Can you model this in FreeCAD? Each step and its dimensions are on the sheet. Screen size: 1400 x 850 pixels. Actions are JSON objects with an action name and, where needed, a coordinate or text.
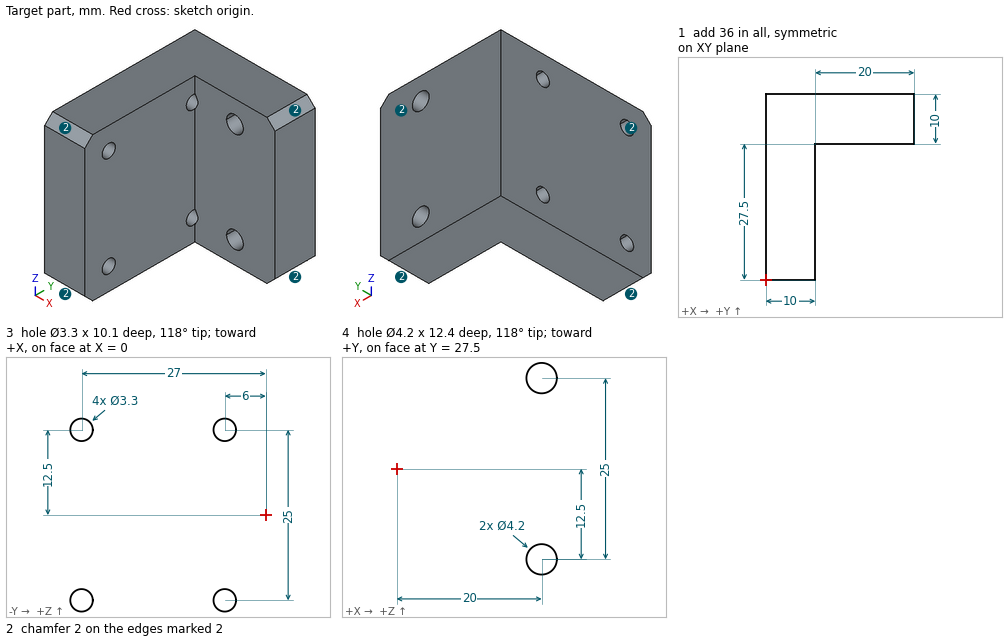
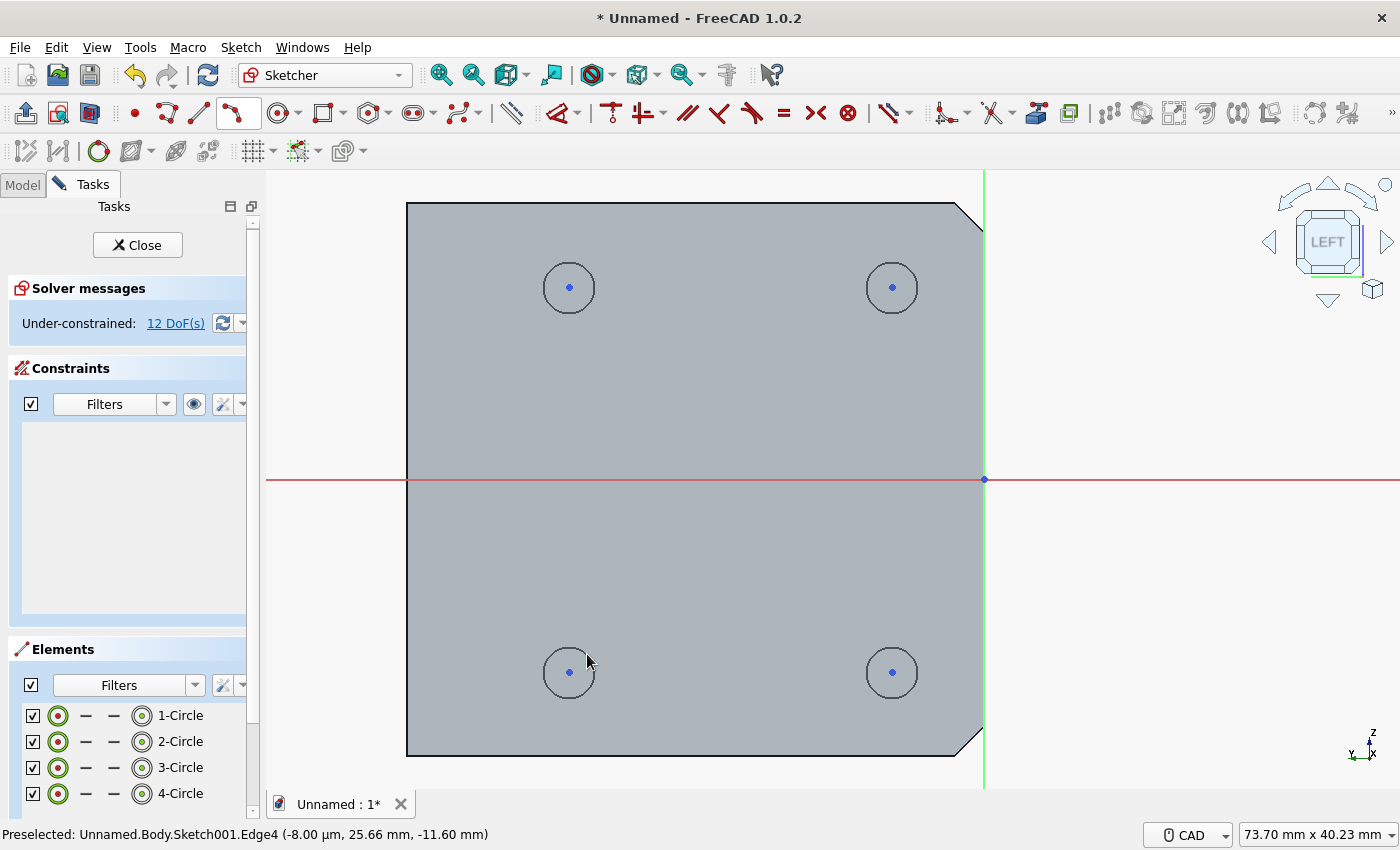
{"action": "left_click", "coordinate": [587, 270]}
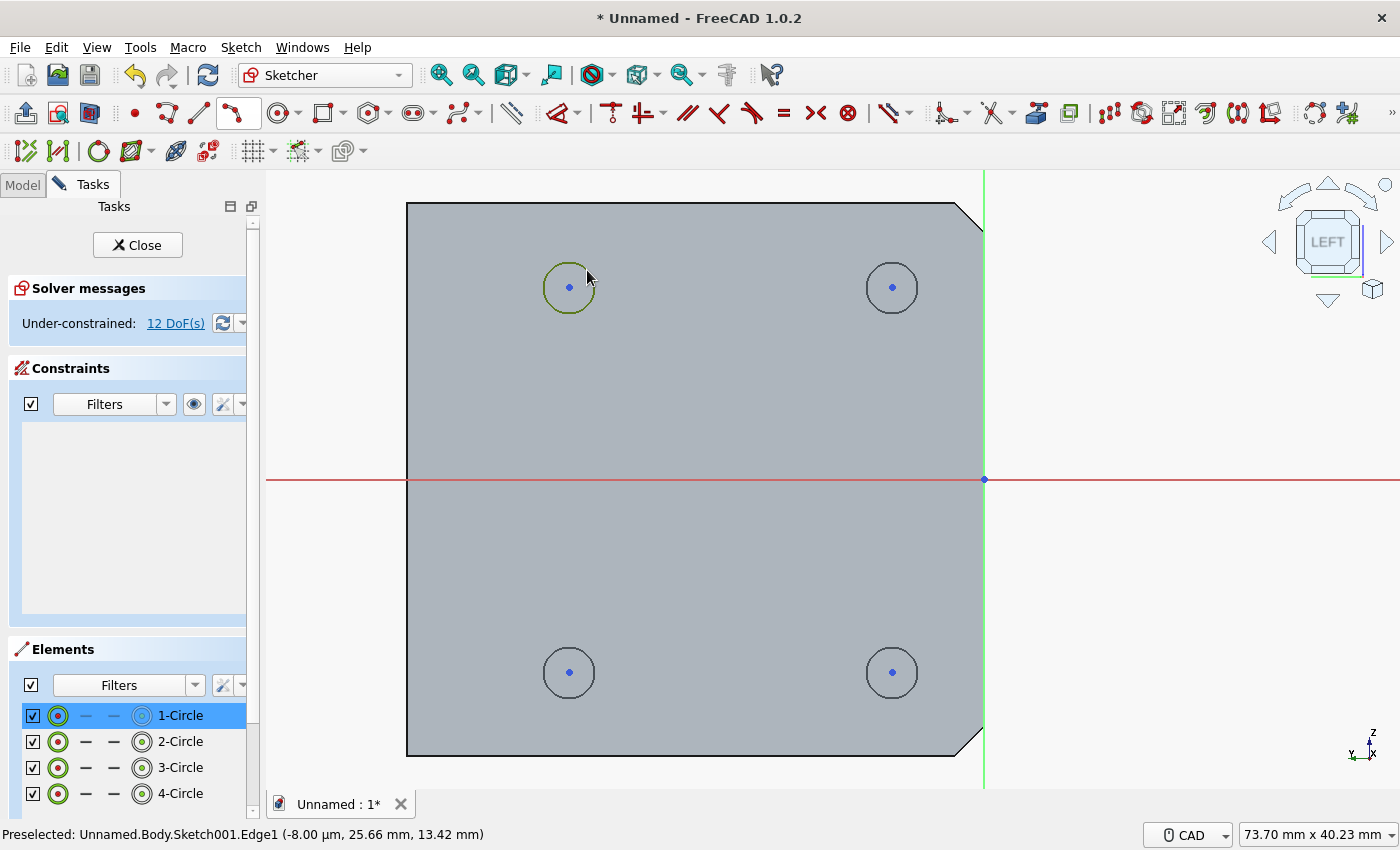
{"action": "left_click", "coordinate": [910, 270]}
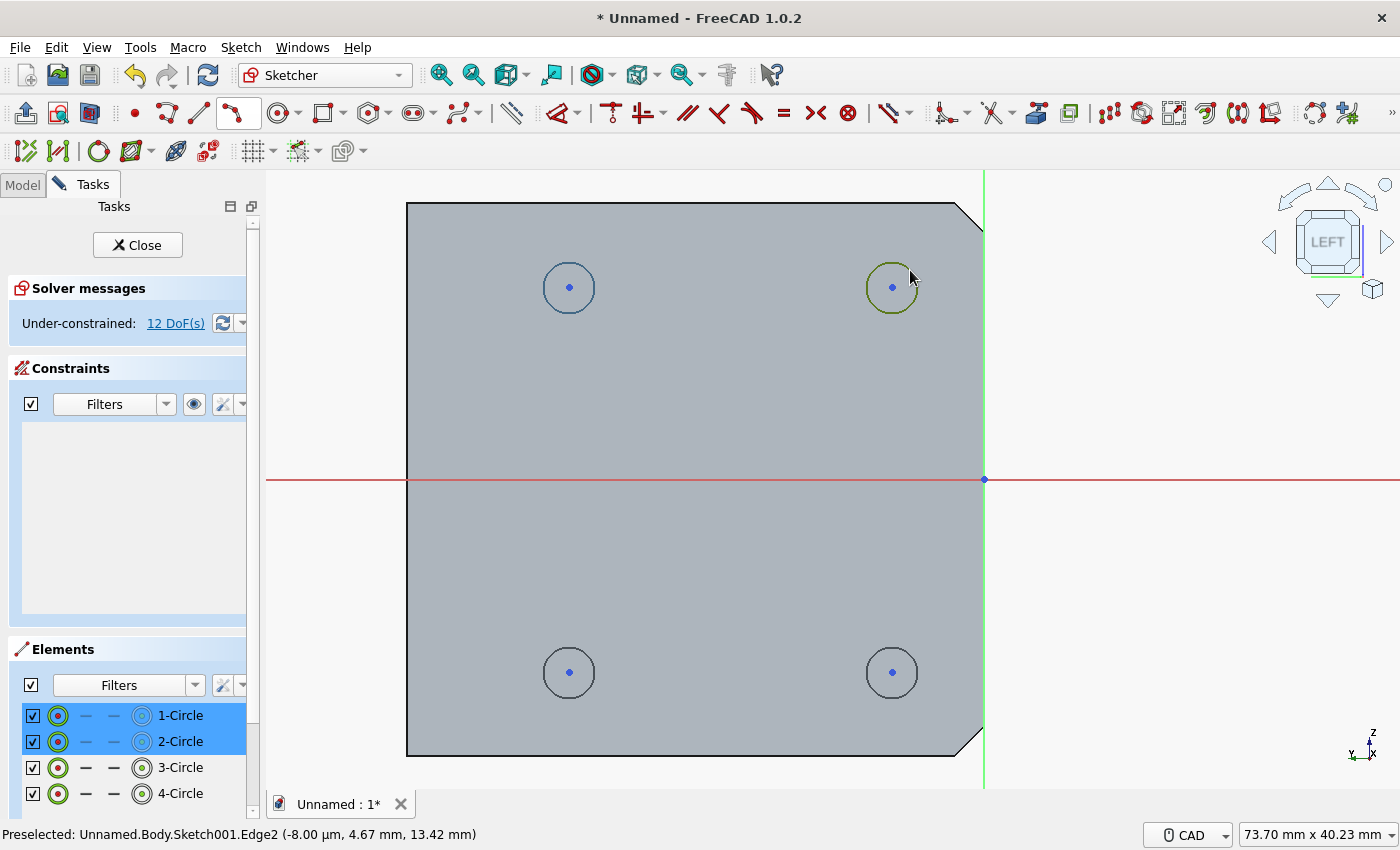
{"action": "left_click", "coordinate": [910, 655]}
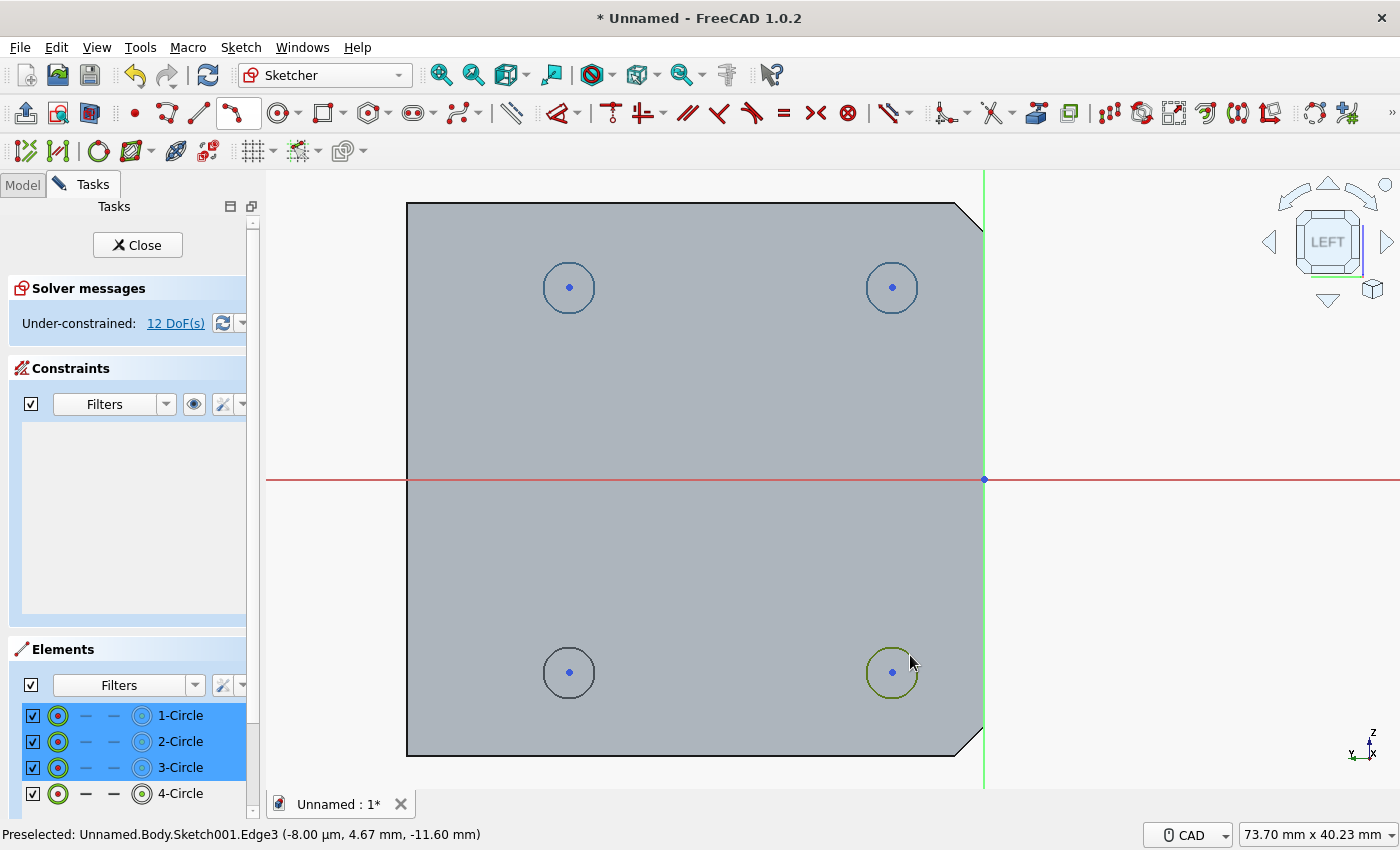
{"action": "left_click", "coordinate": [587, 655]}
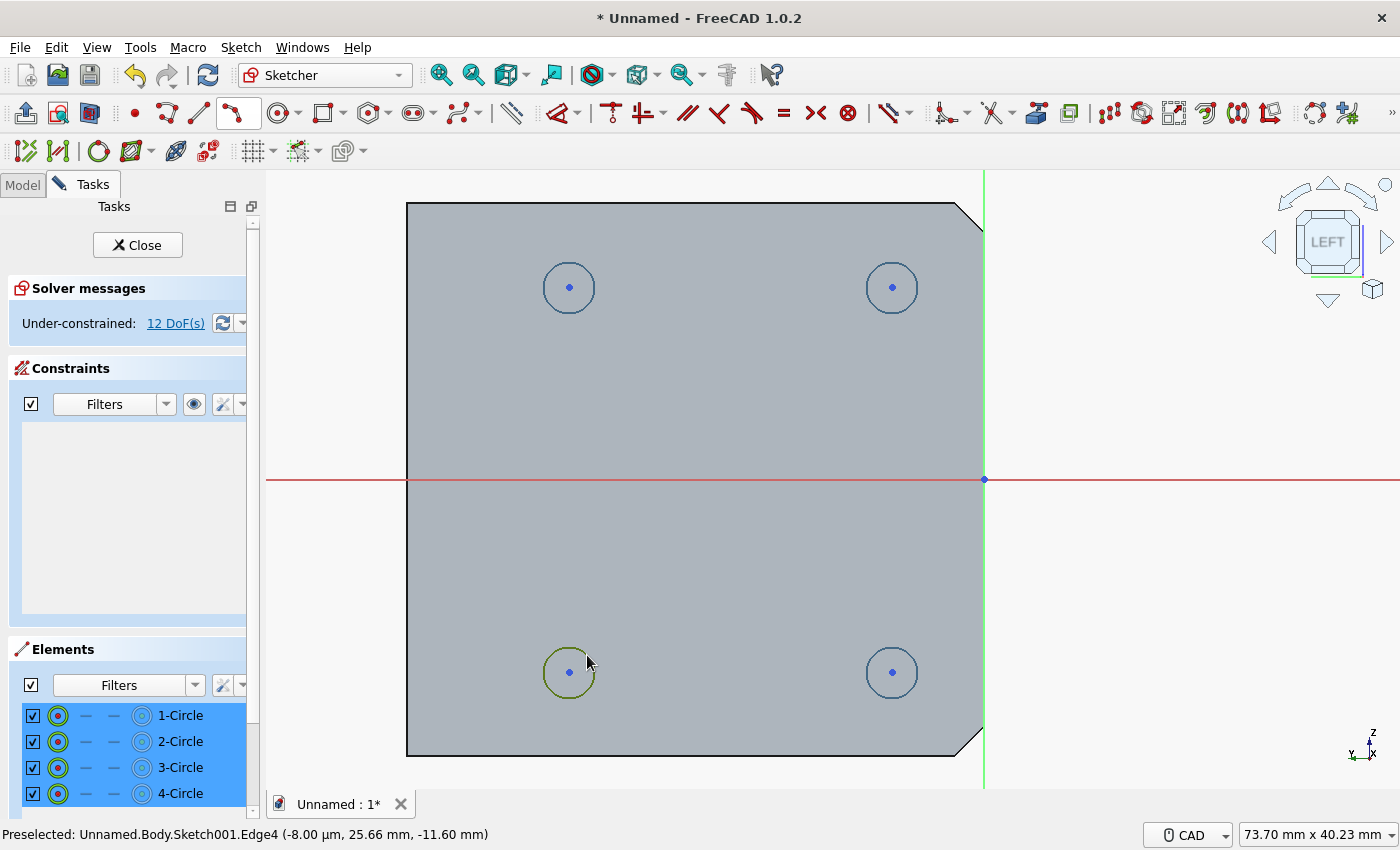
{"action": "key", "text": "e"}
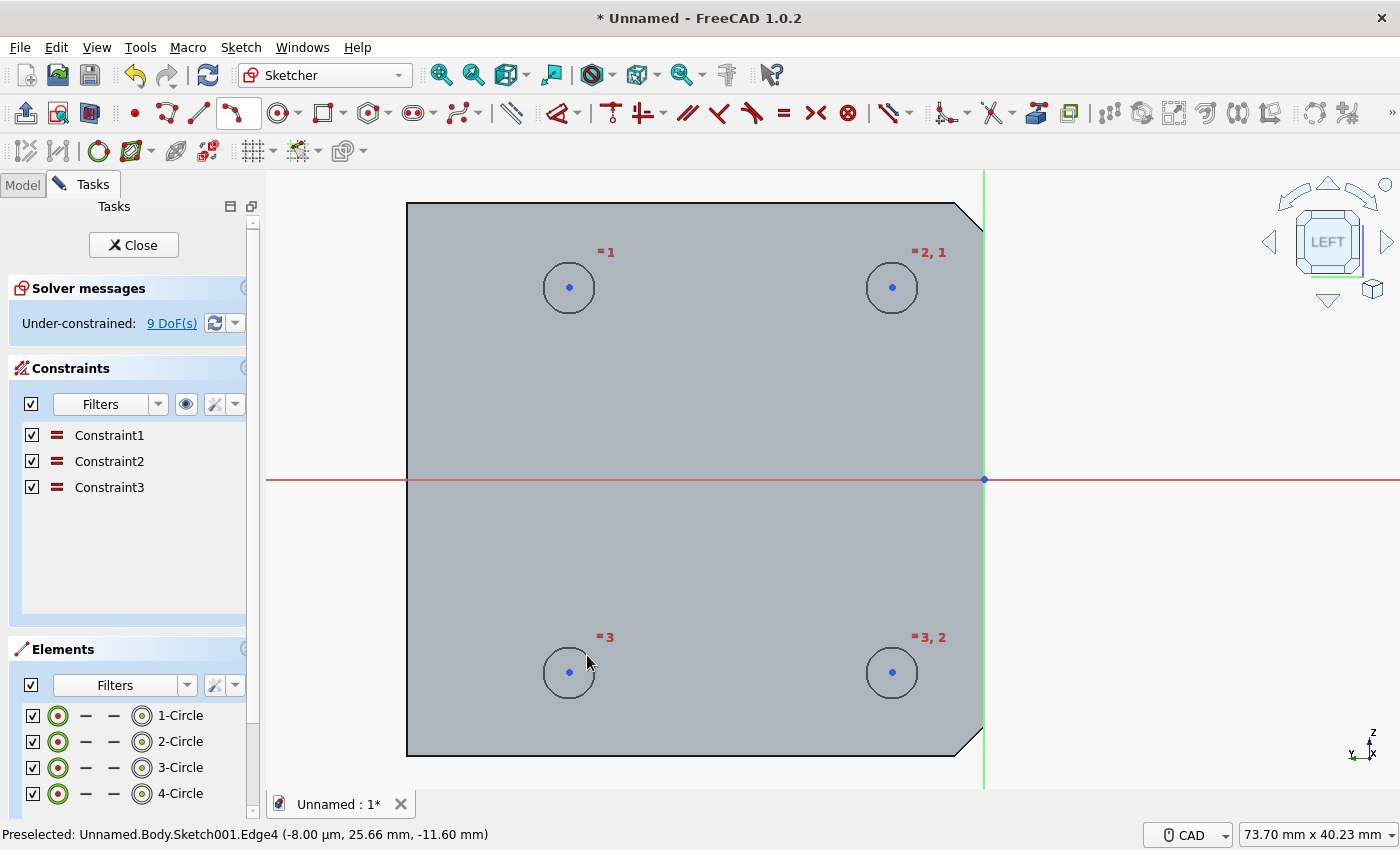
{"action": "left_click", "coordinate": [569, 288]}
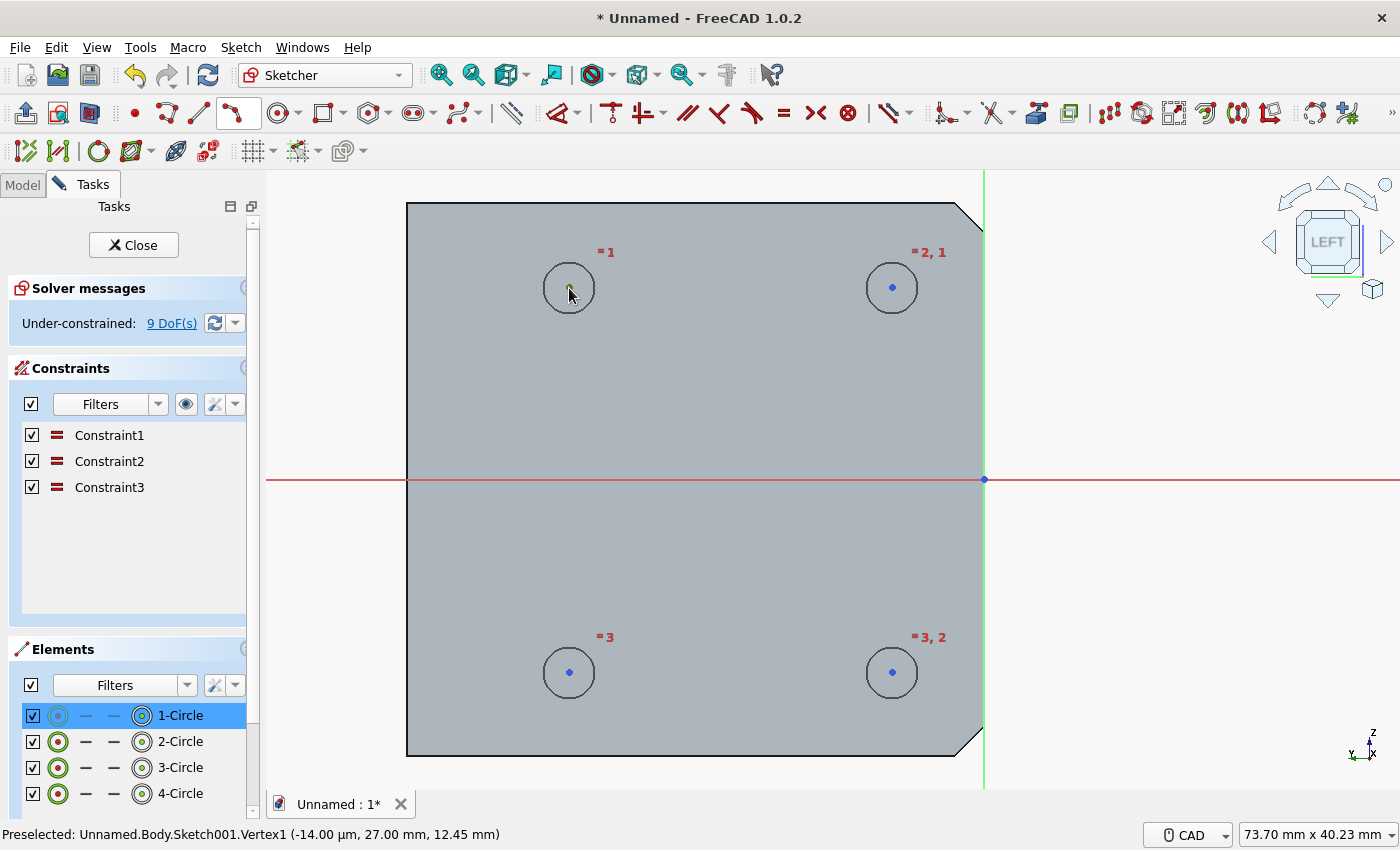
{"action": "left_click", "coordinate": [892, 288]}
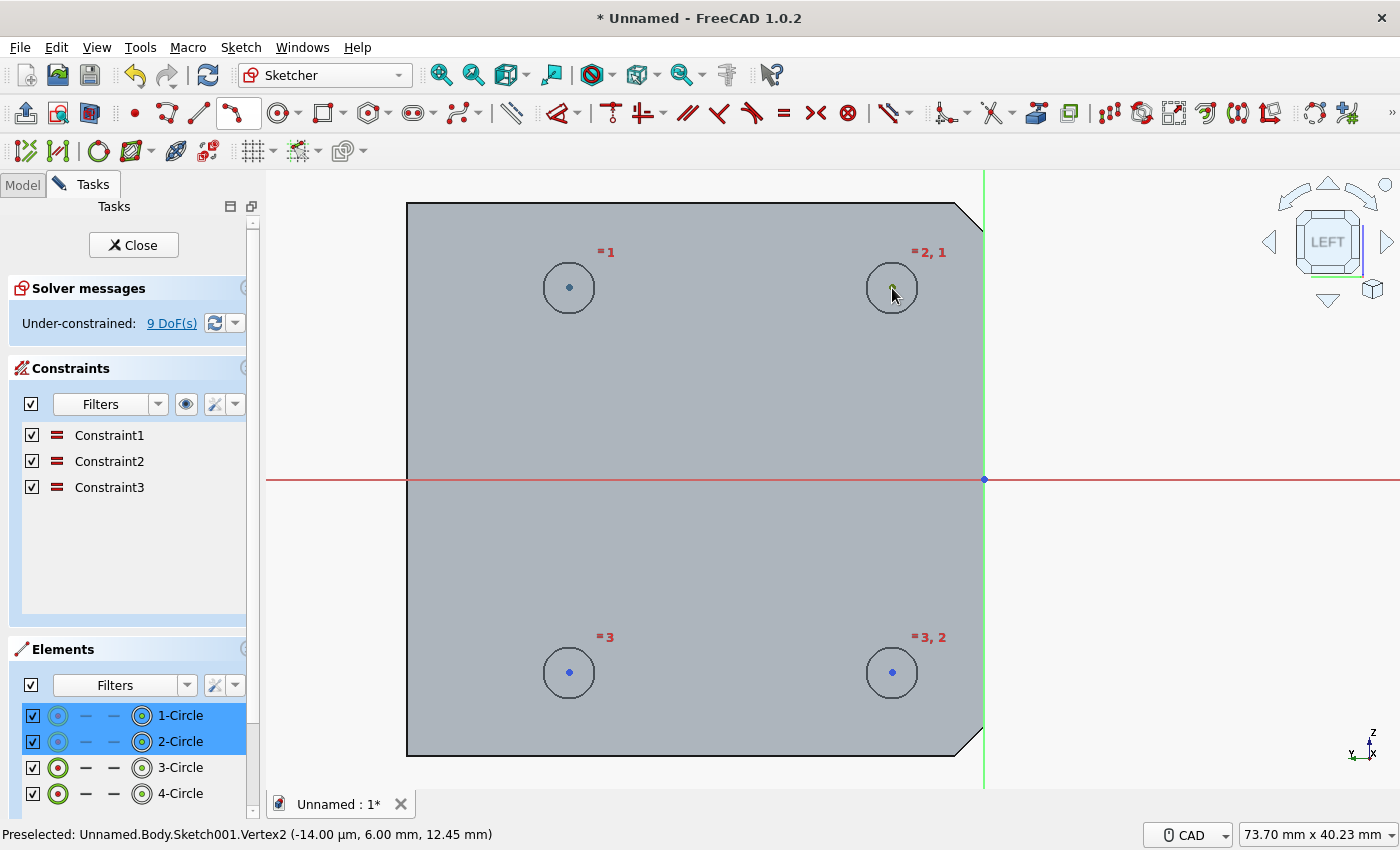
{"action": "key", "text": "h"}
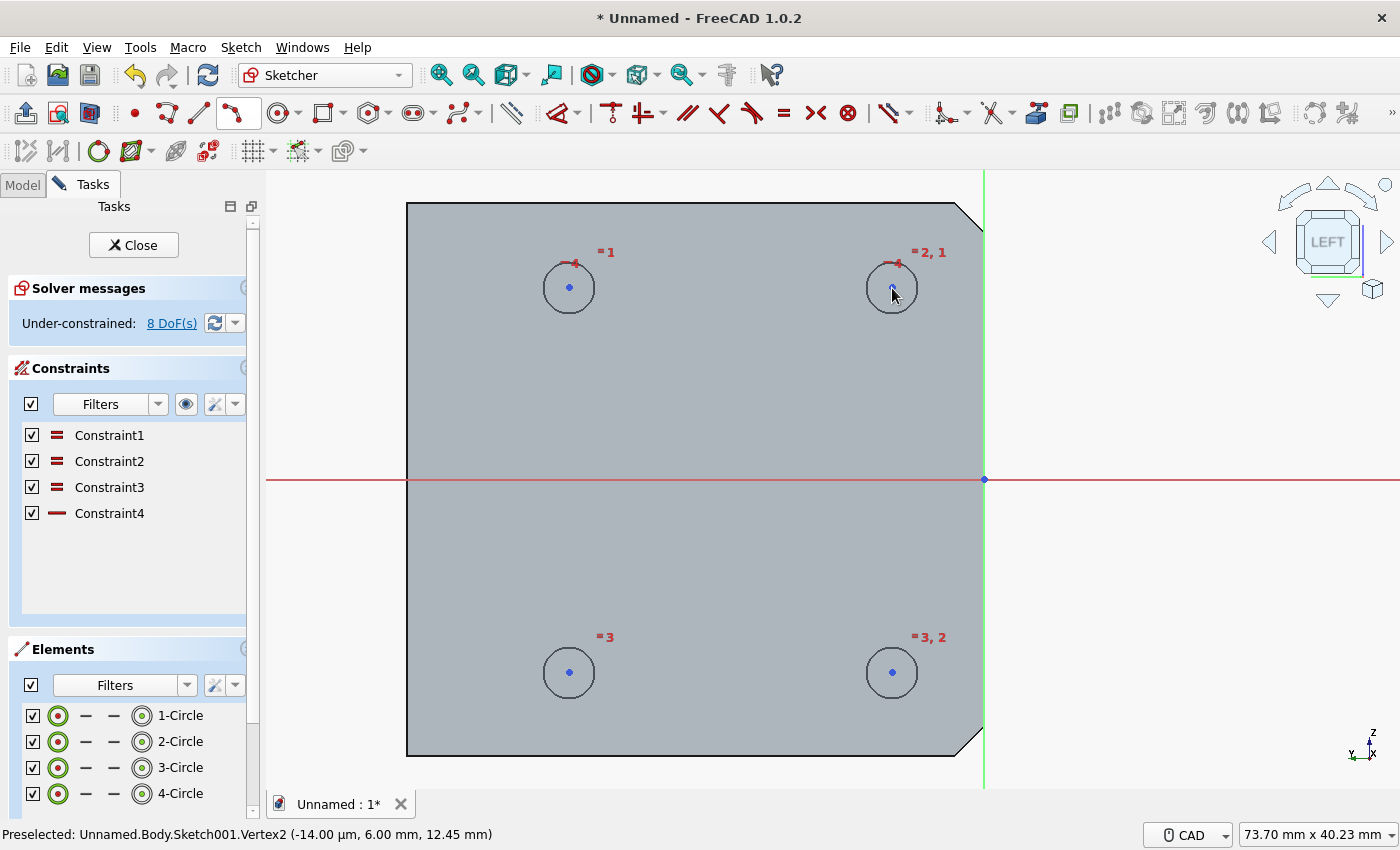
{"action": "left_click", "coordinate": [892, 288]}